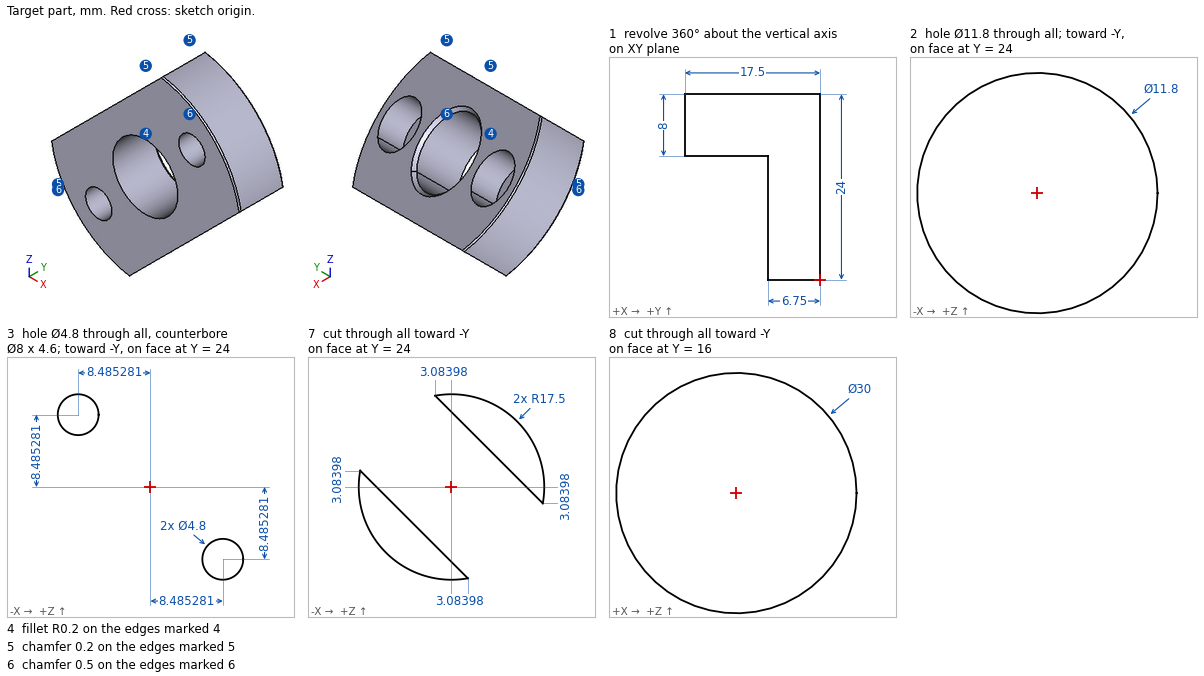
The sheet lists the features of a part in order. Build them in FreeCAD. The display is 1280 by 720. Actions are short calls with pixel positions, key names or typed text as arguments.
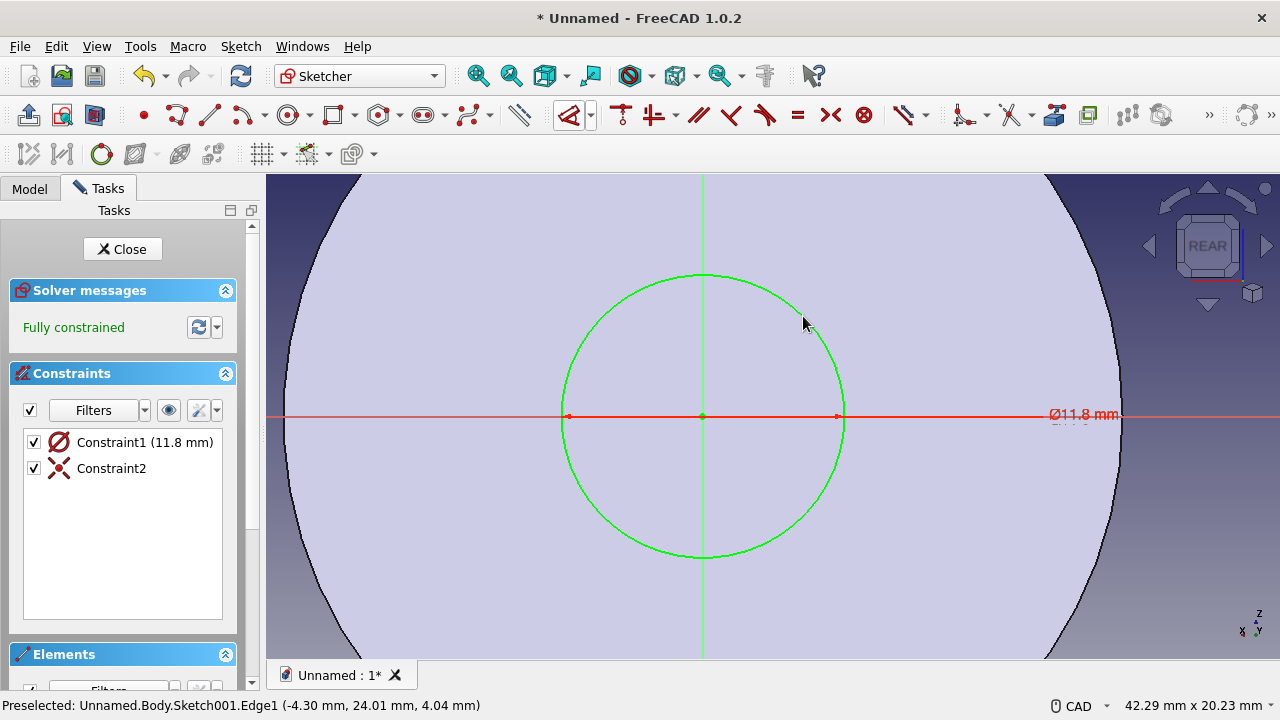
click(123, 249)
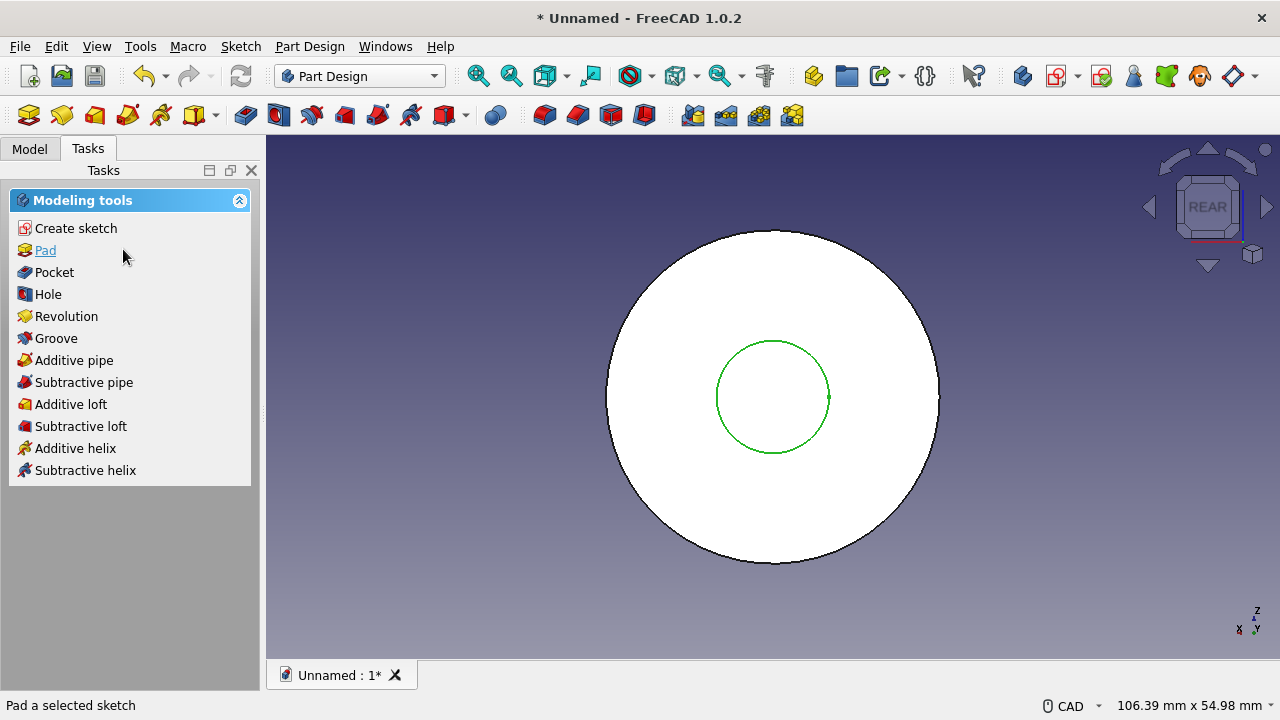
click(279, 116)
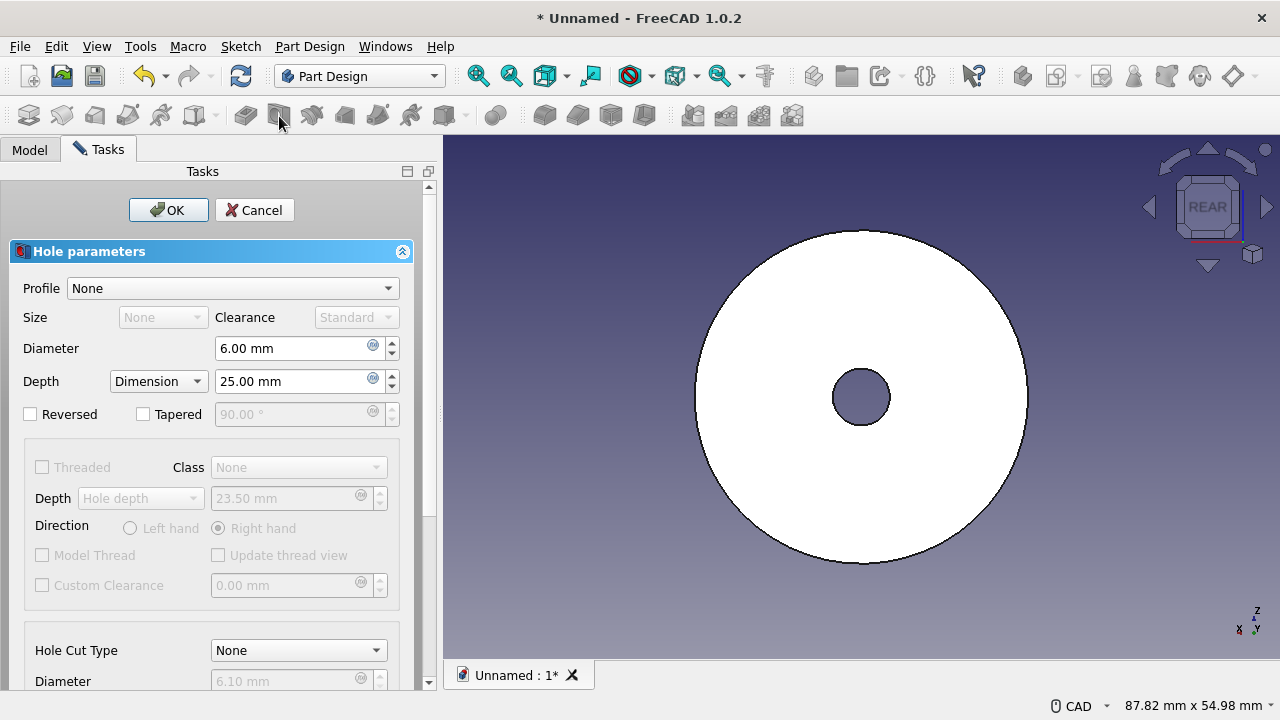
triple_click(300, 348)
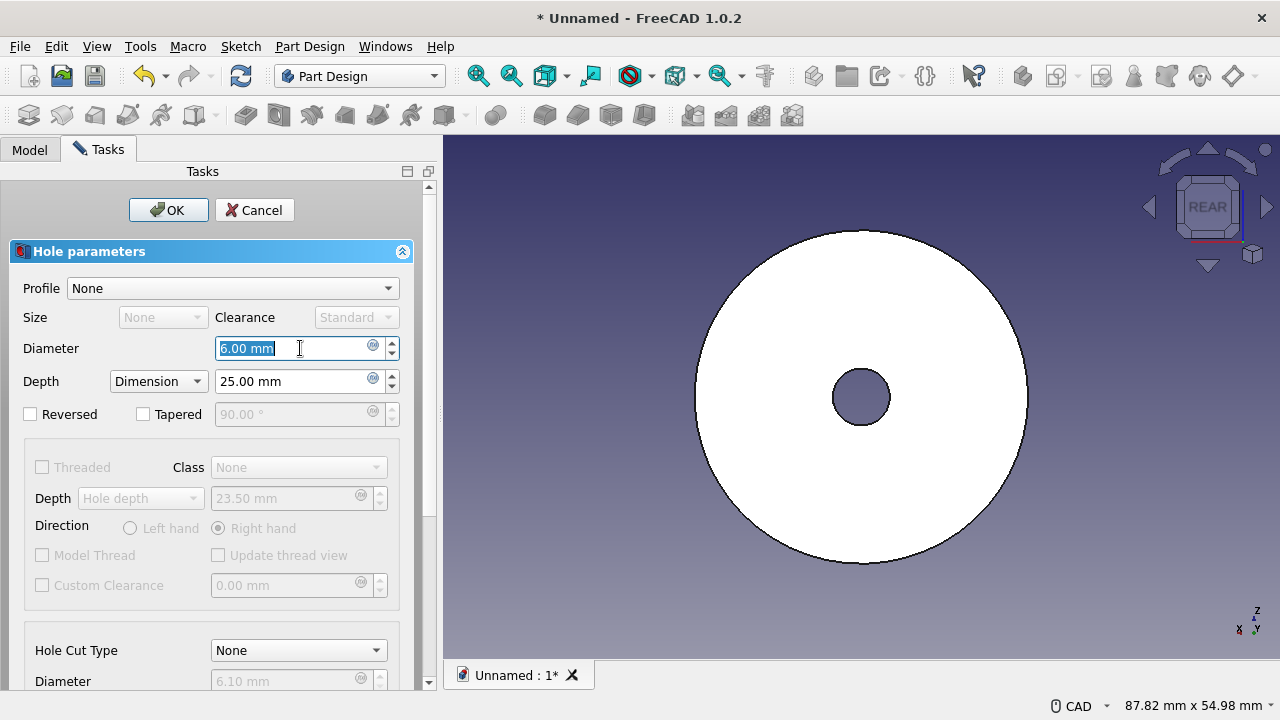
text(11.8)
key(Tab)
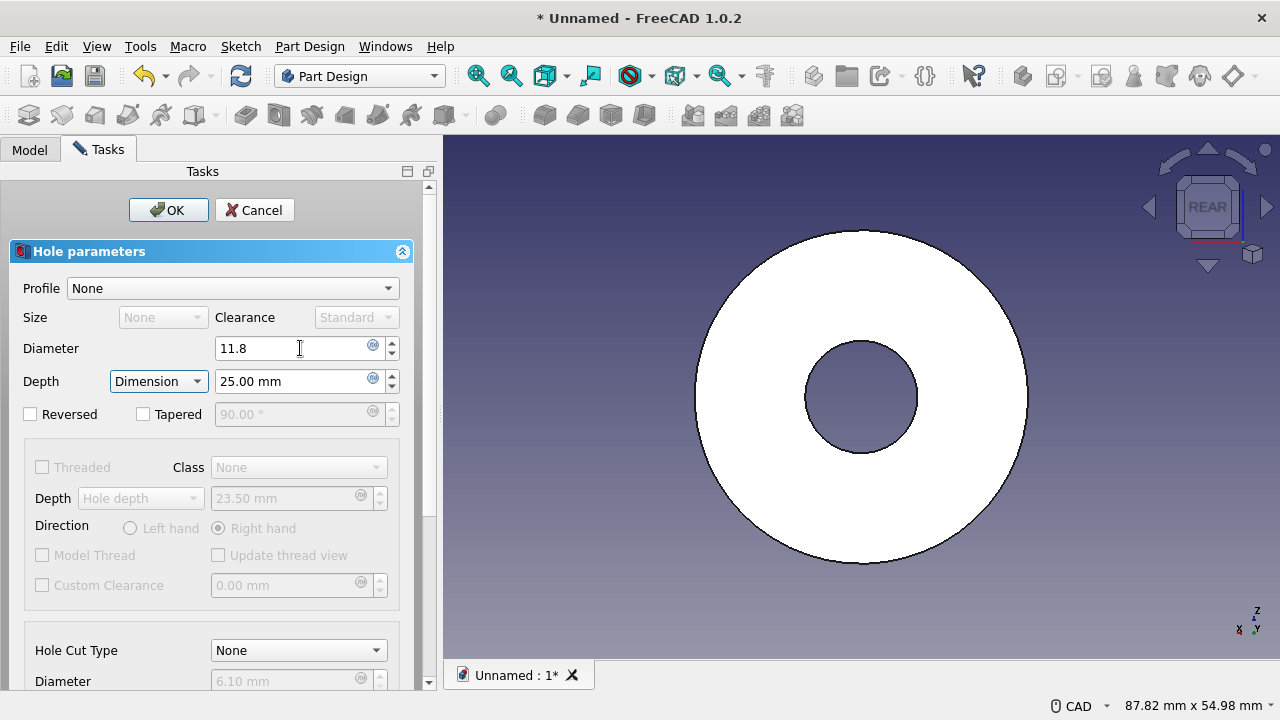
click(160, 382)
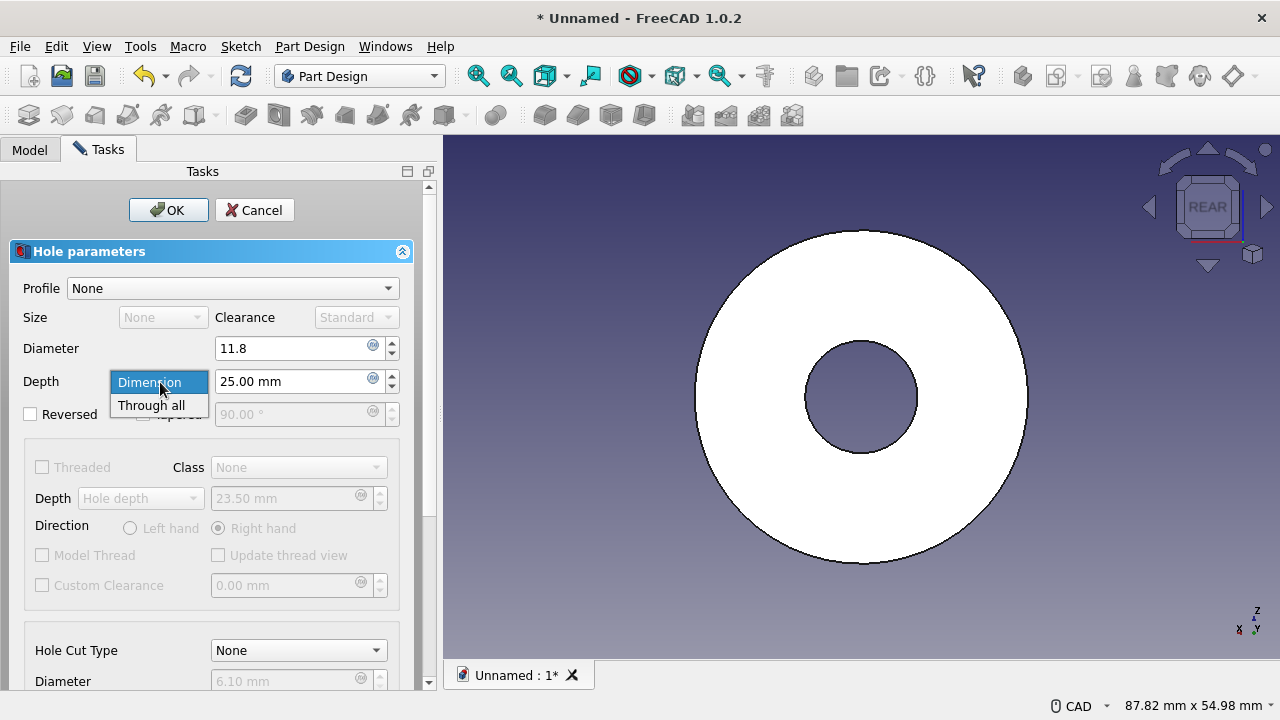
click(158, 406)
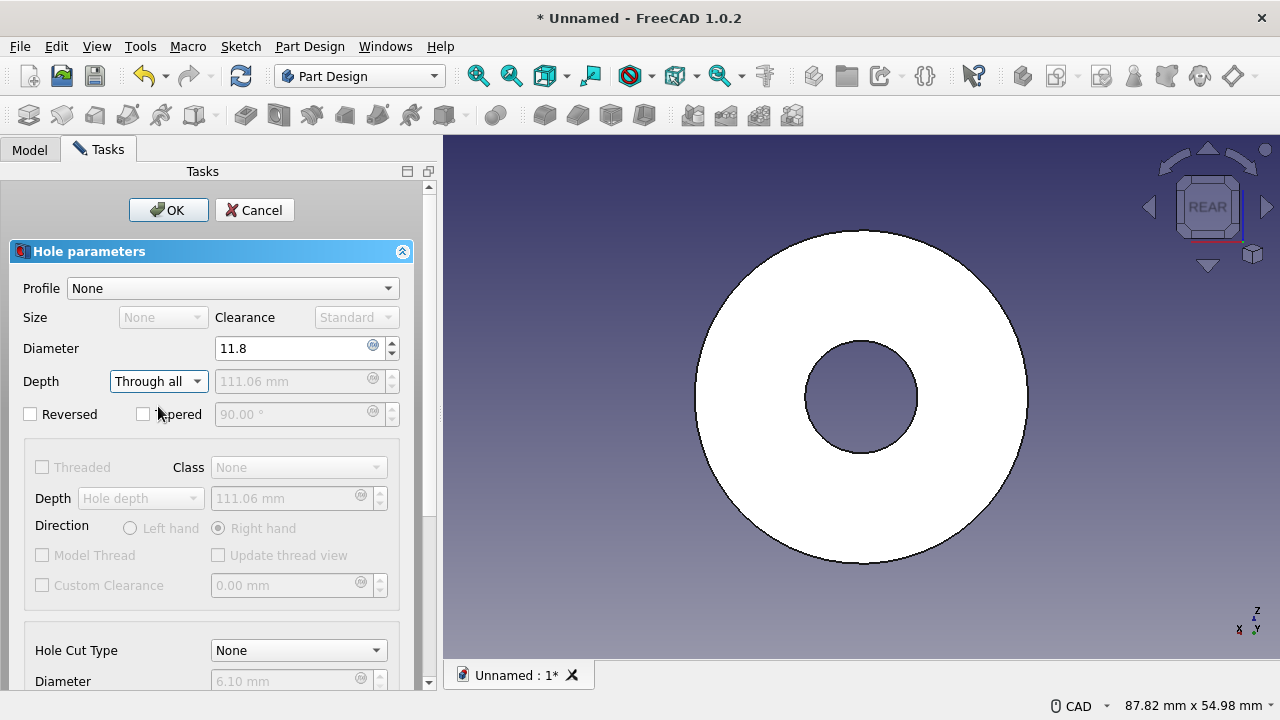
click(169, 210)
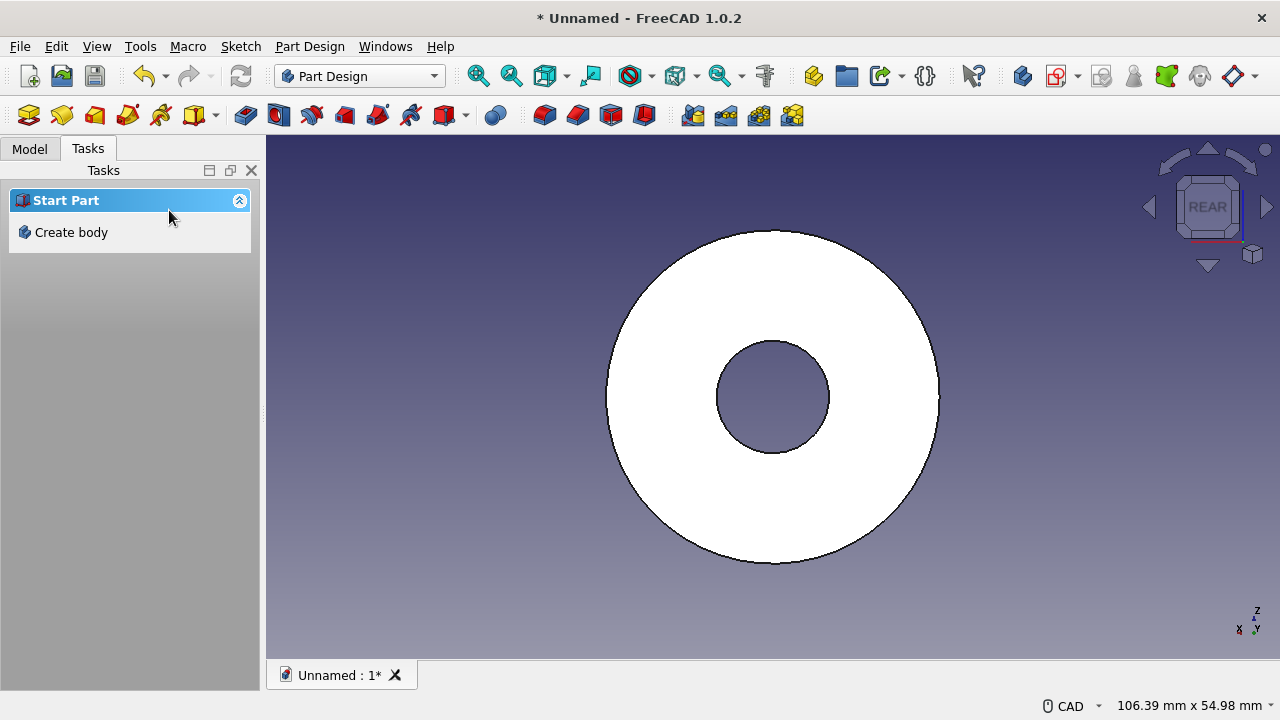
click(725, 301)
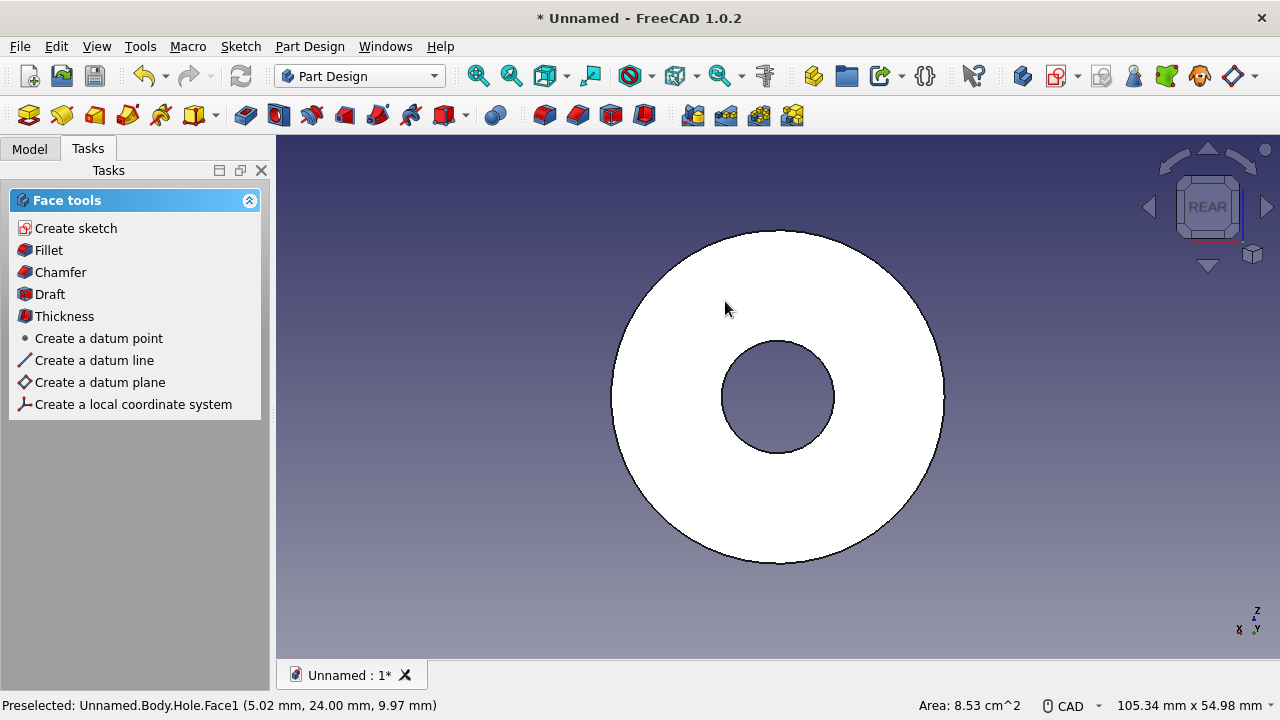
click(1056, 76)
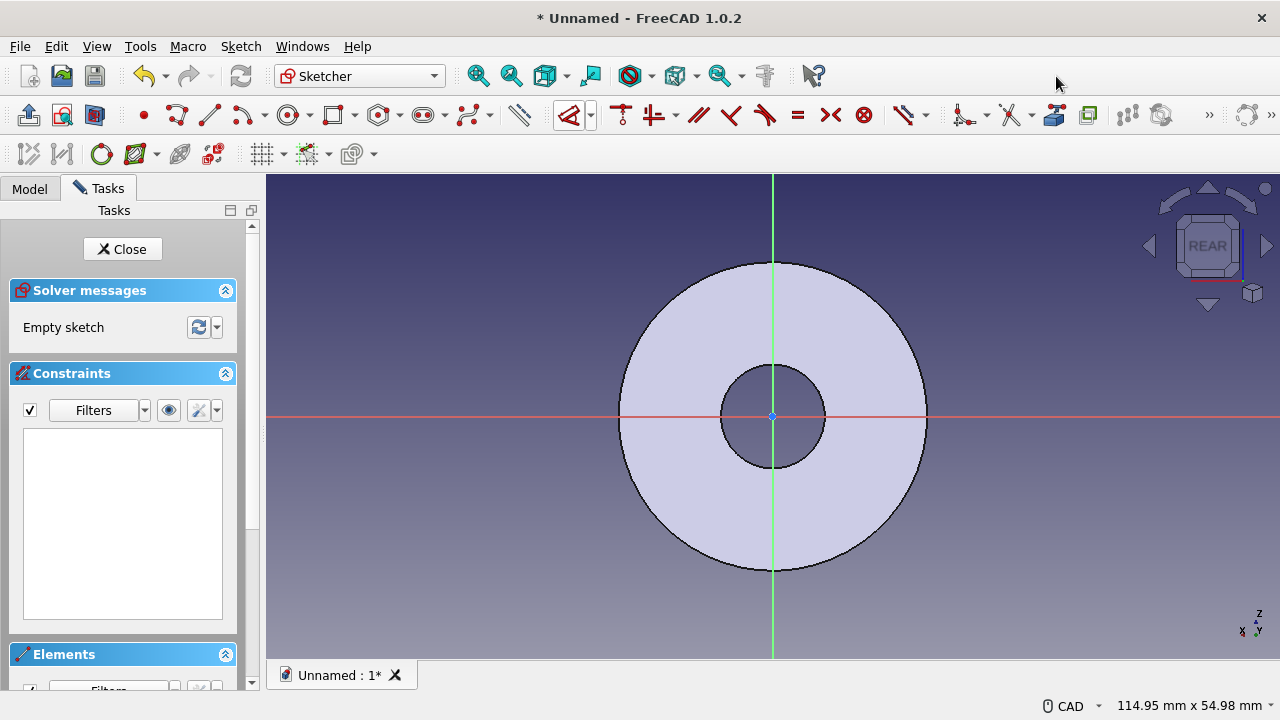
scroll(912, 417, up, 2)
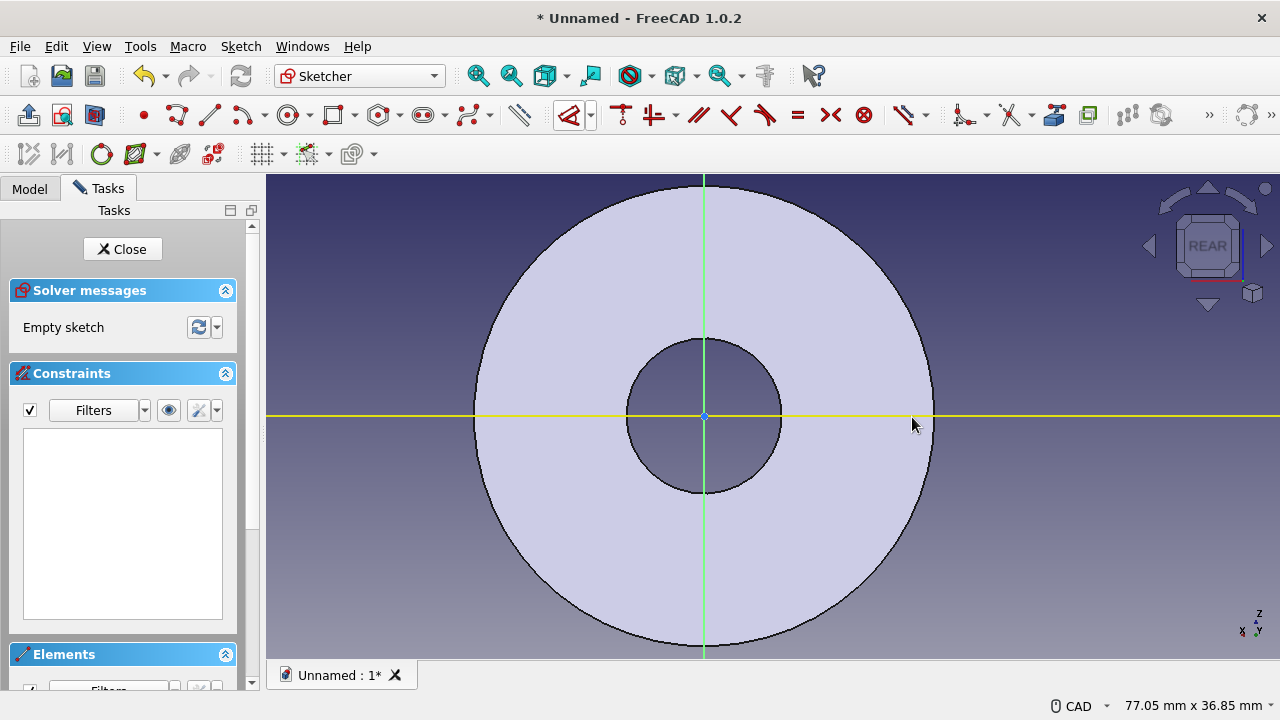
click(288, 116)